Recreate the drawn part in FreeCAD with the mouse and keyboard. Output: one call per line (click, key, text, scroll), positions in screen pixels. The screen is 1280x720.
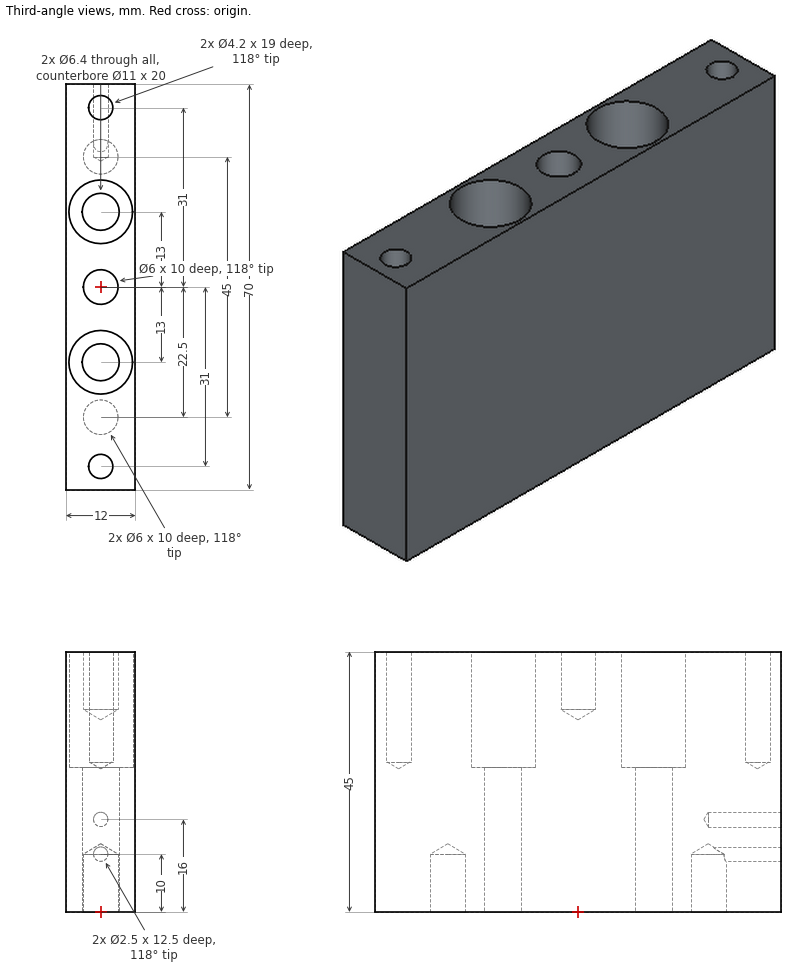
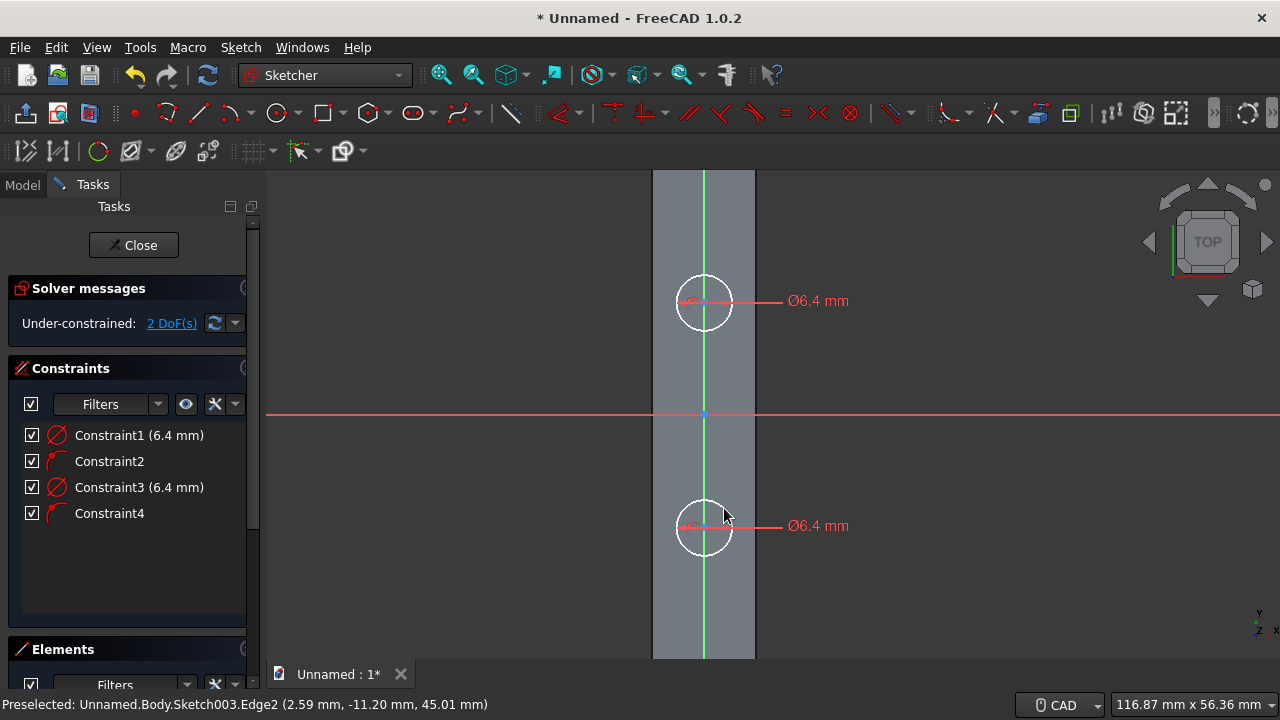
click(558, 114)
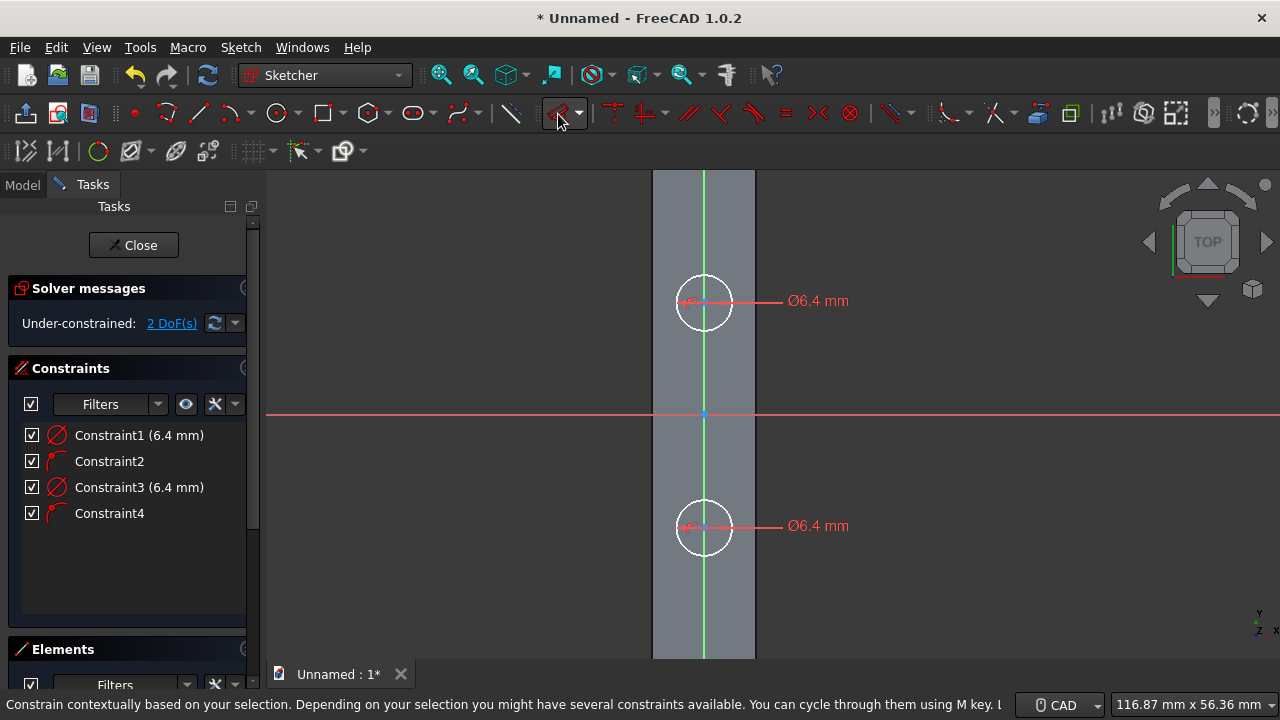
click(704, 303)
click(738, 359)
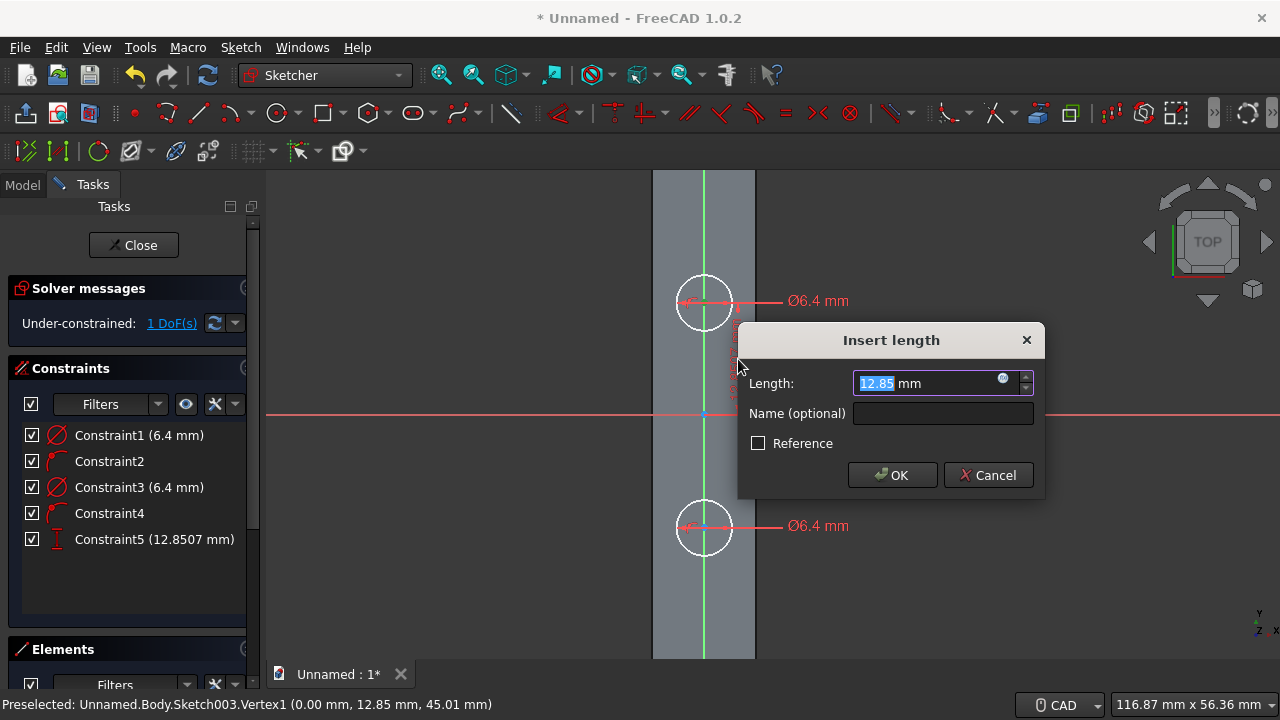
text(13)
key(Return)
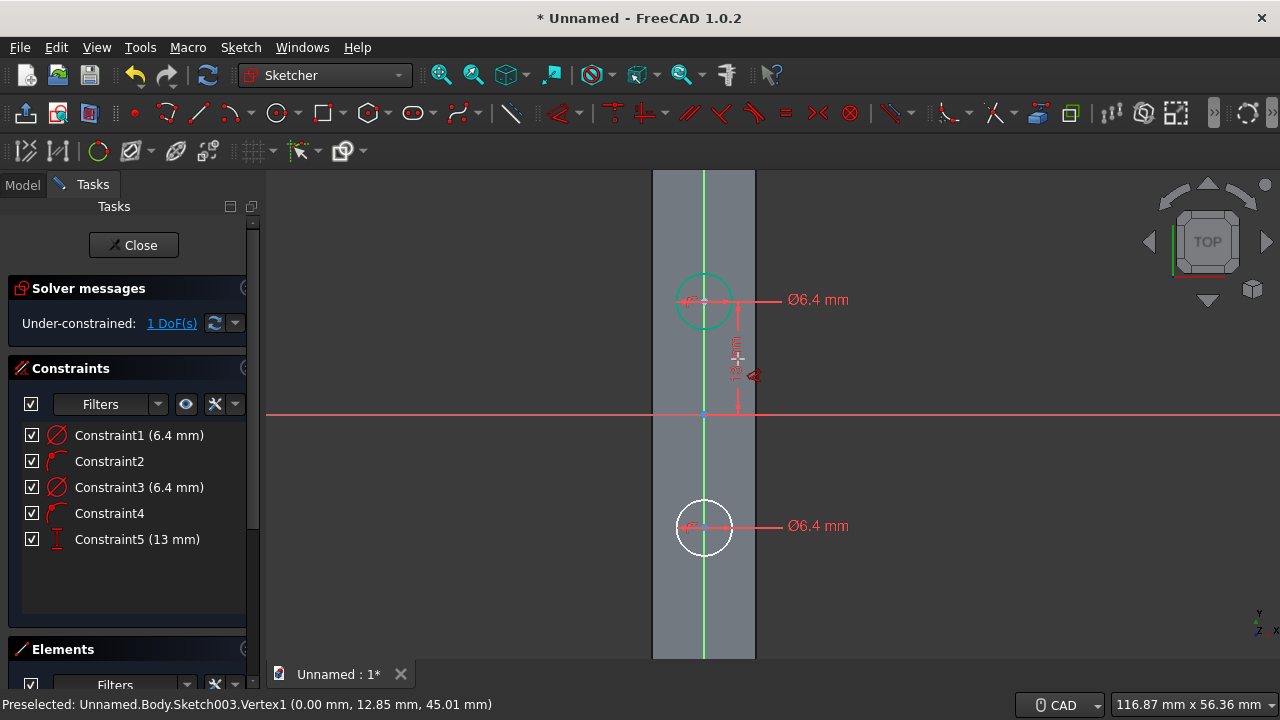
click(704, 528)
click(738, 471)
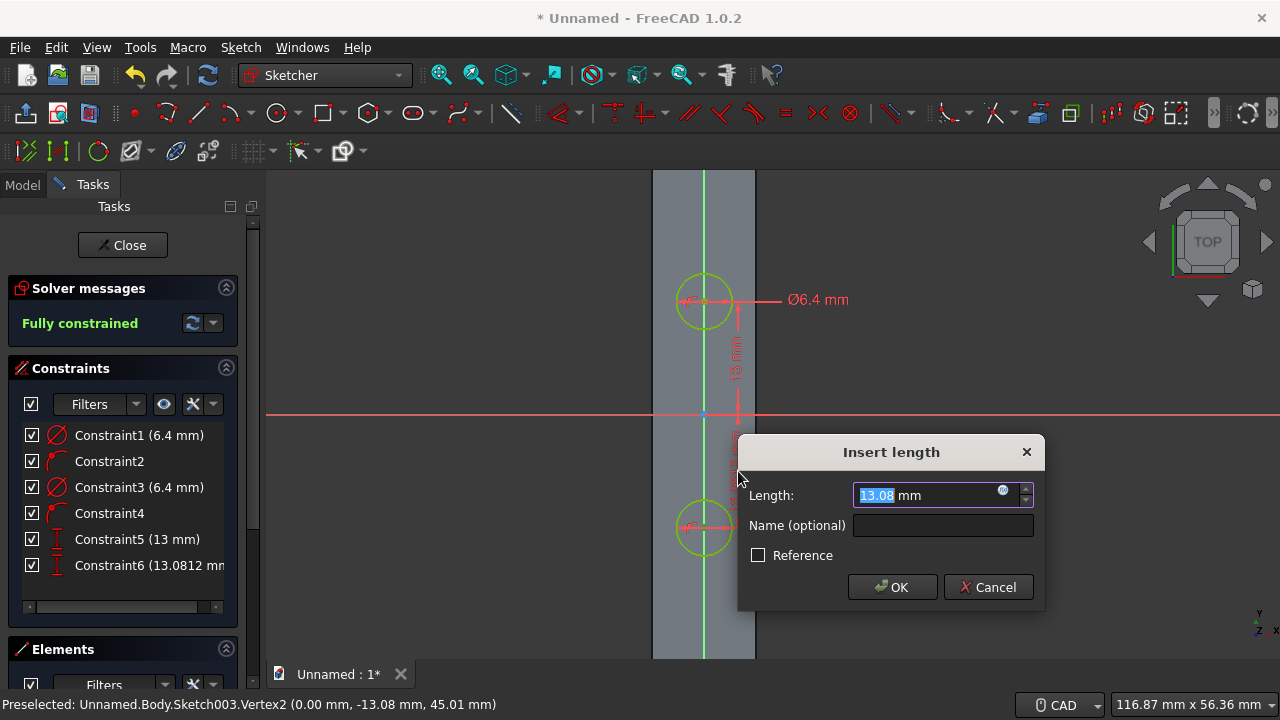
text(13)
key(Return)
key(Escape)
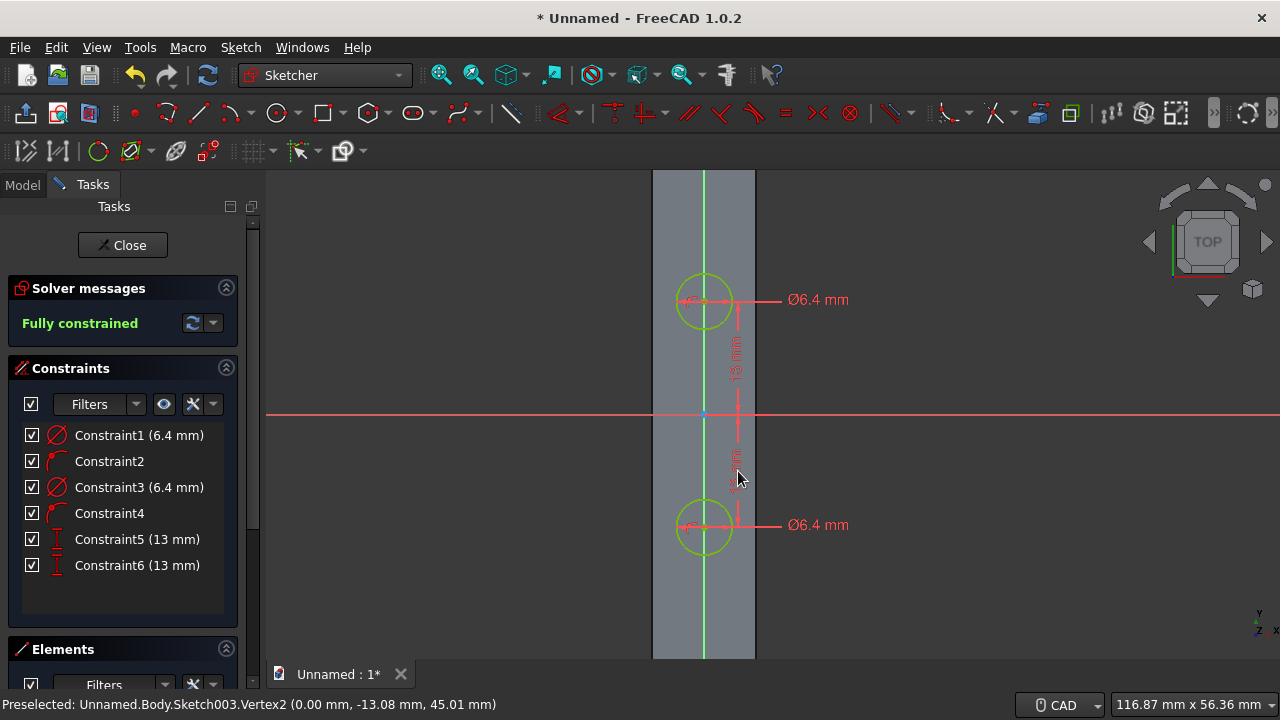
click(123, 245)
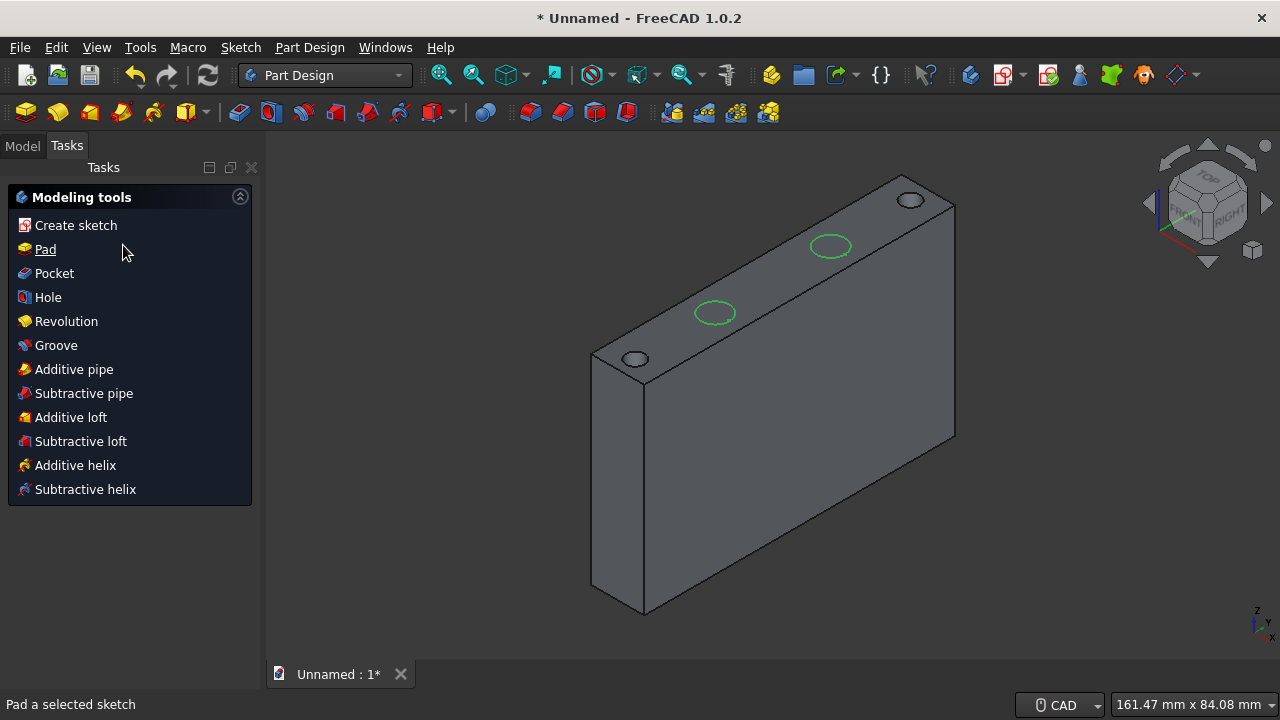
click(272, 112)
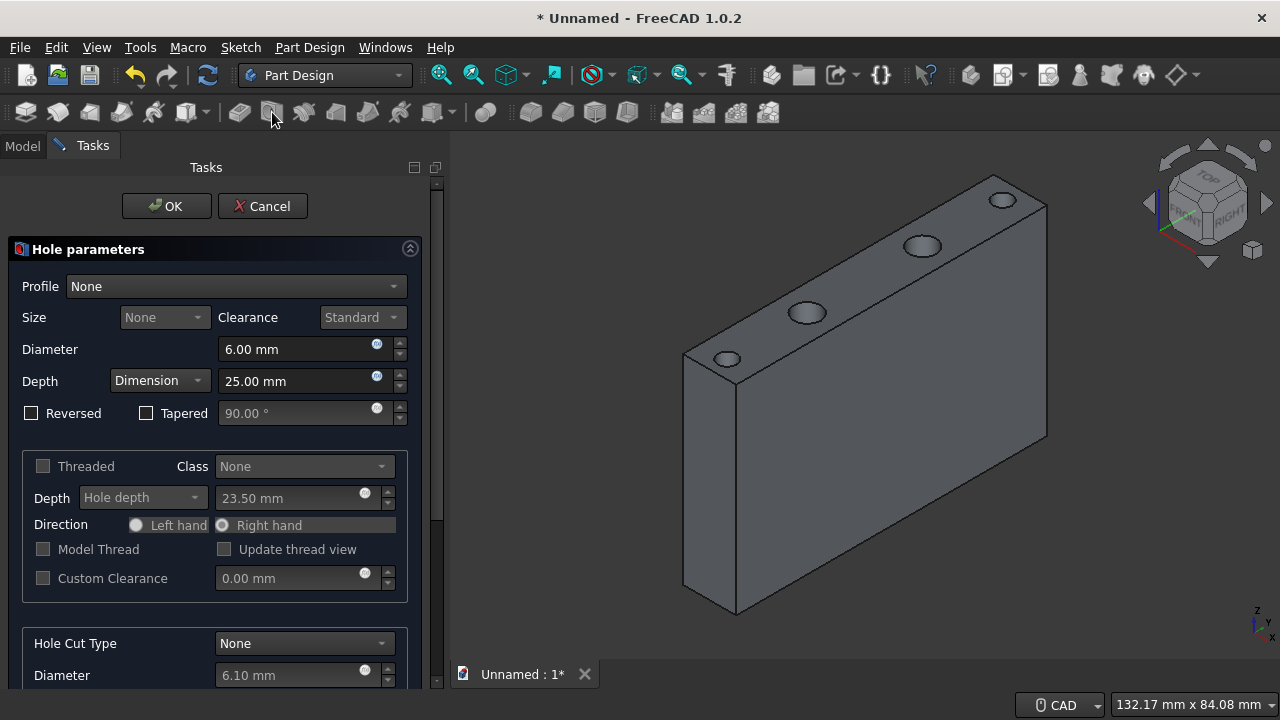
triple_click(305, 349)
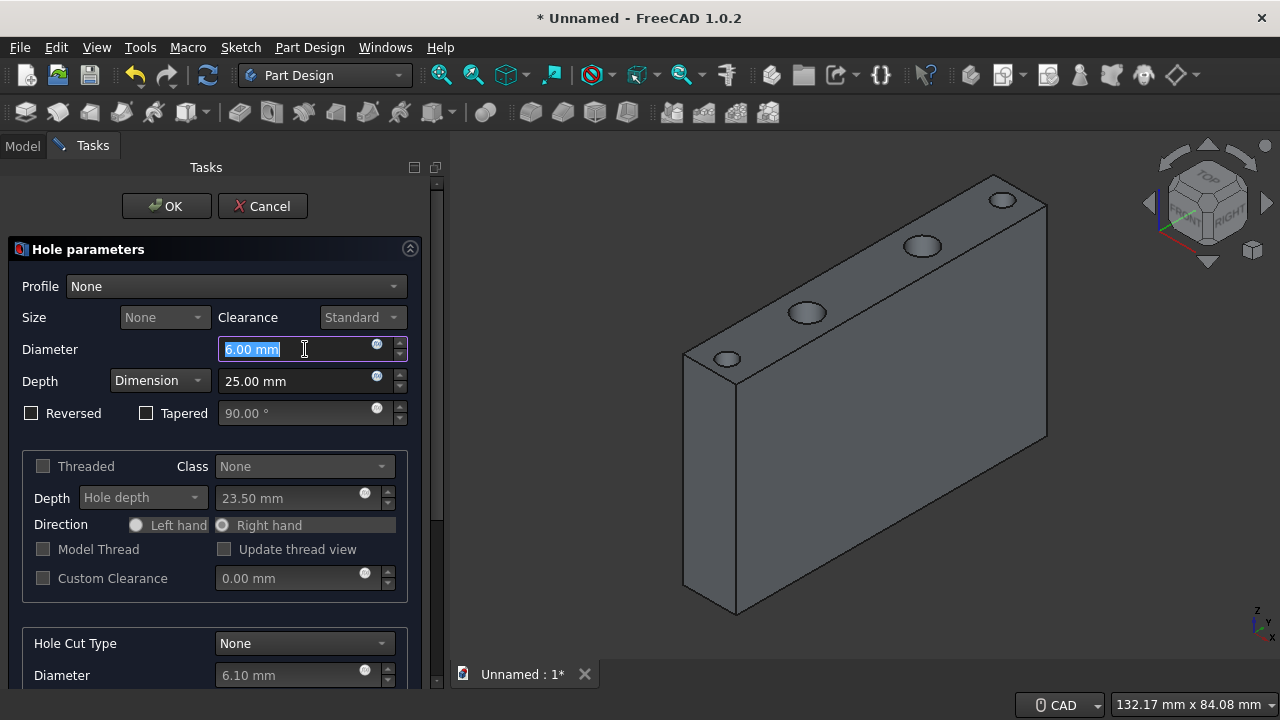
text(6.4)
key(Tab)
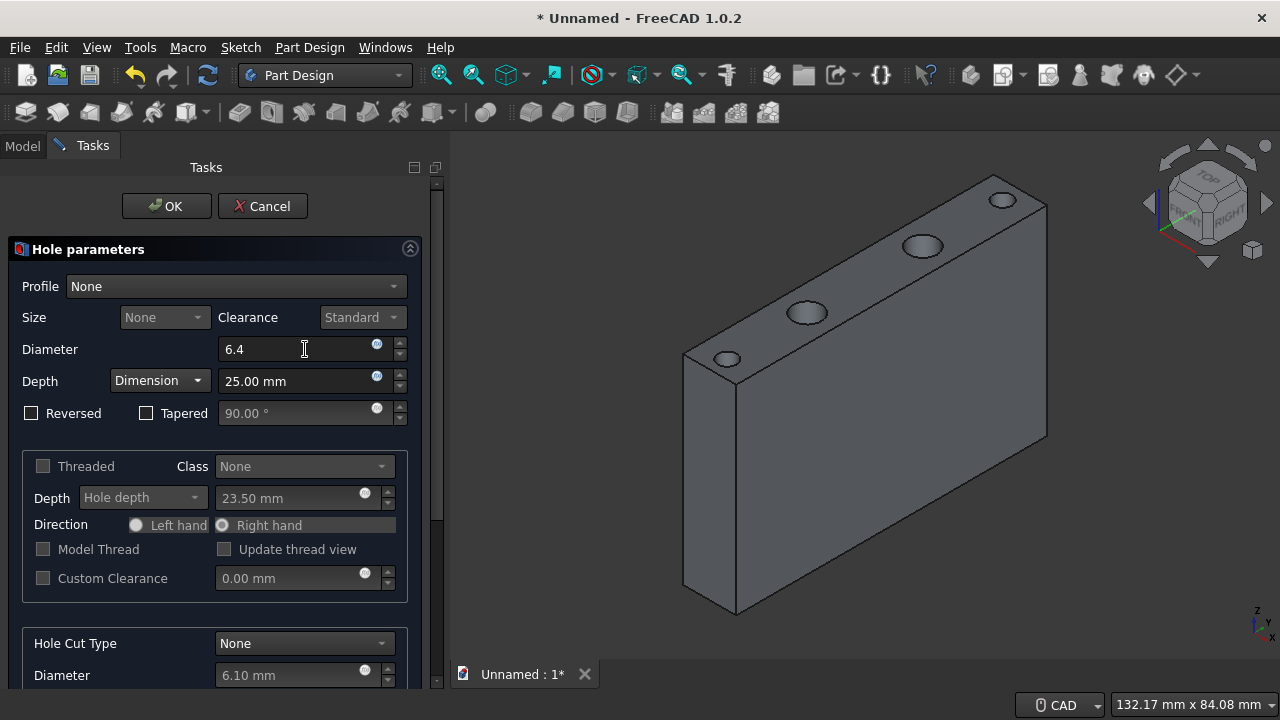
click(161, 380)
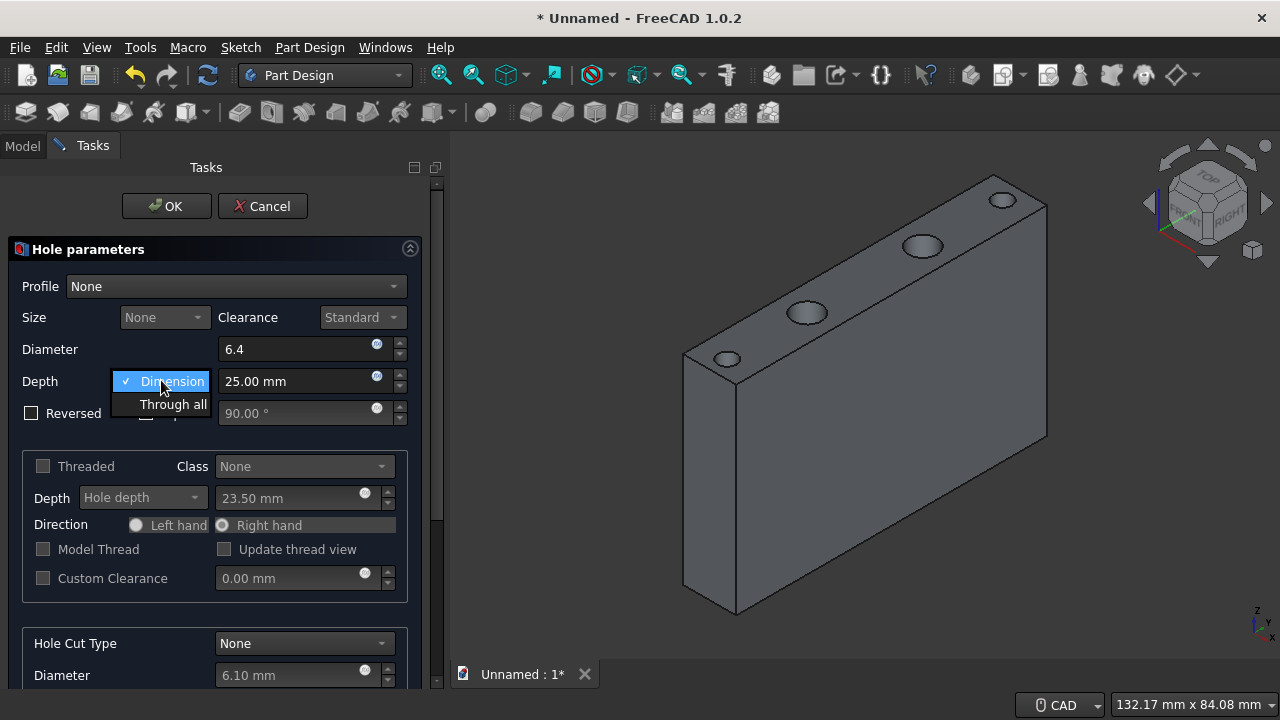
click(160, 404)